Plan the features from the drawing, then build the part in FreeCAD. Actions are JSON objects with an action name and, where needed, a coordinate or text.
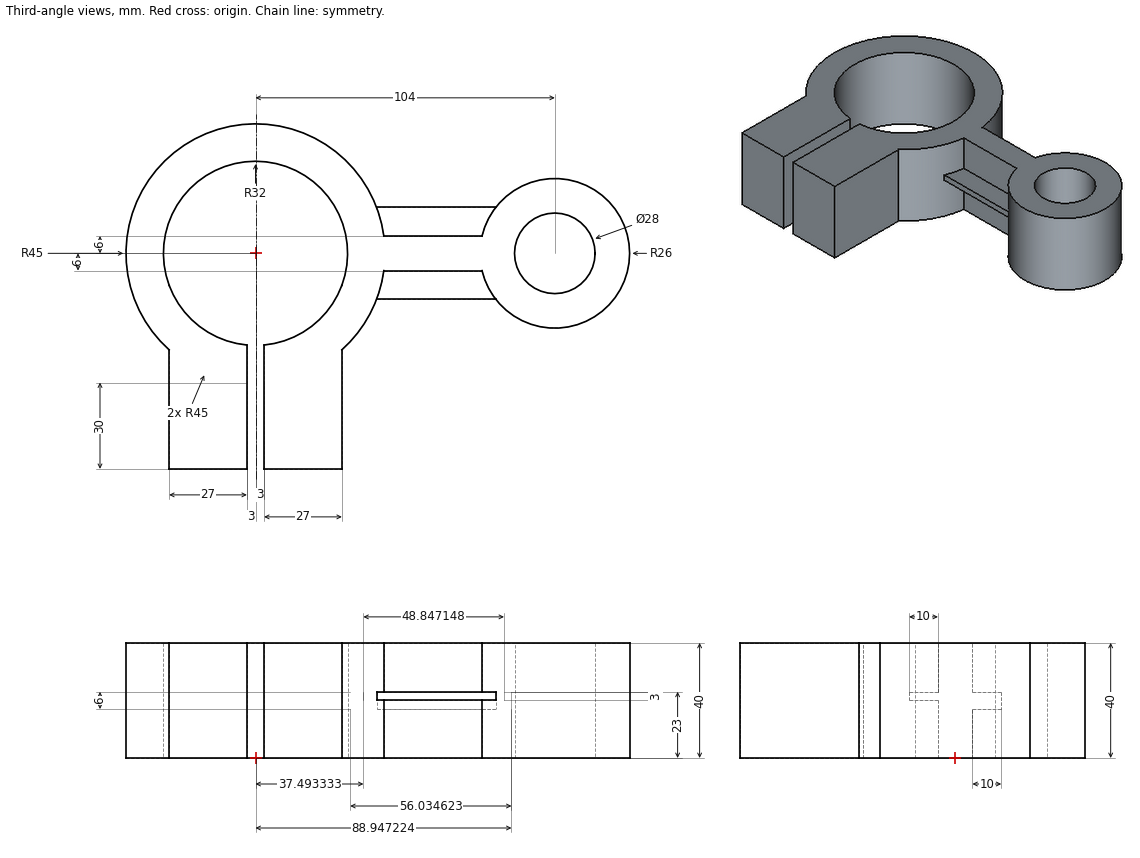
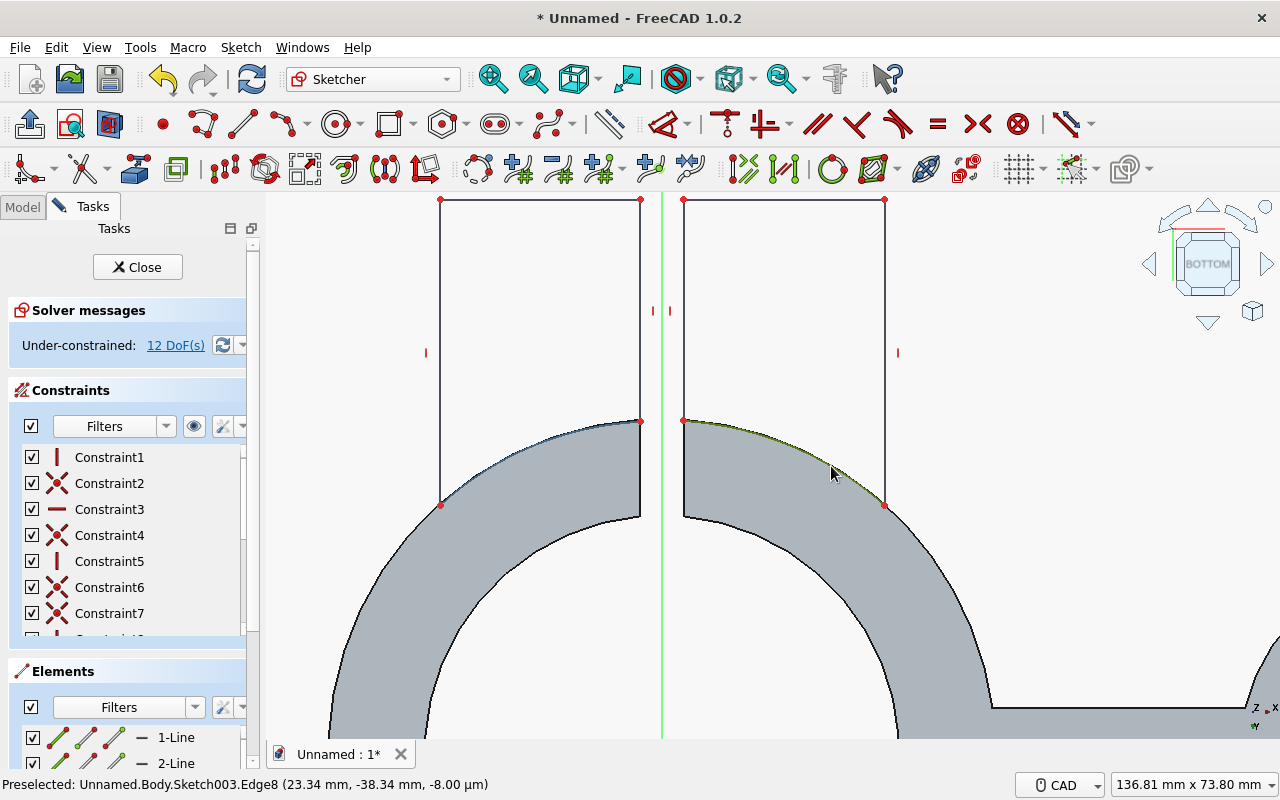
{"action": "left_click", "coordinate": [726, 124]}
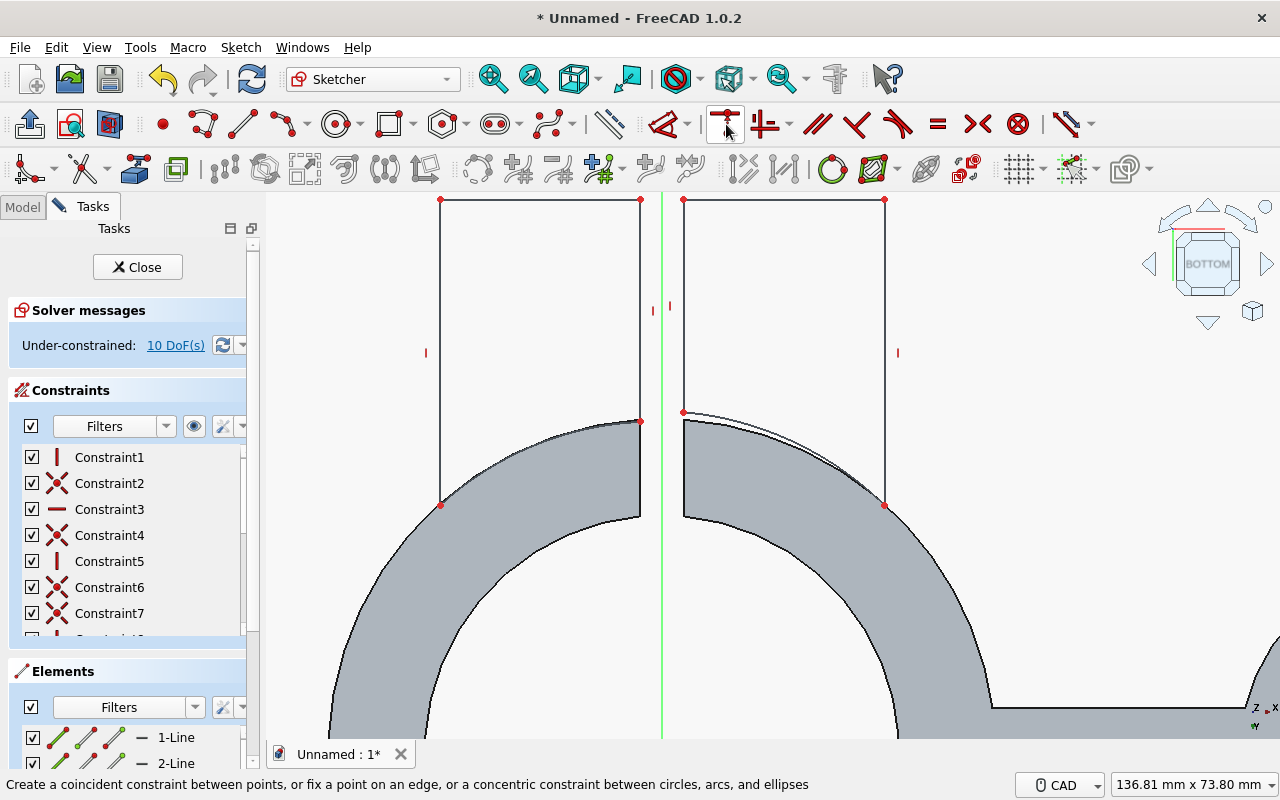
{"action": "scroll", "coordinate": [791, 446], "scroll_direction": "down", "scroll_amount": 2}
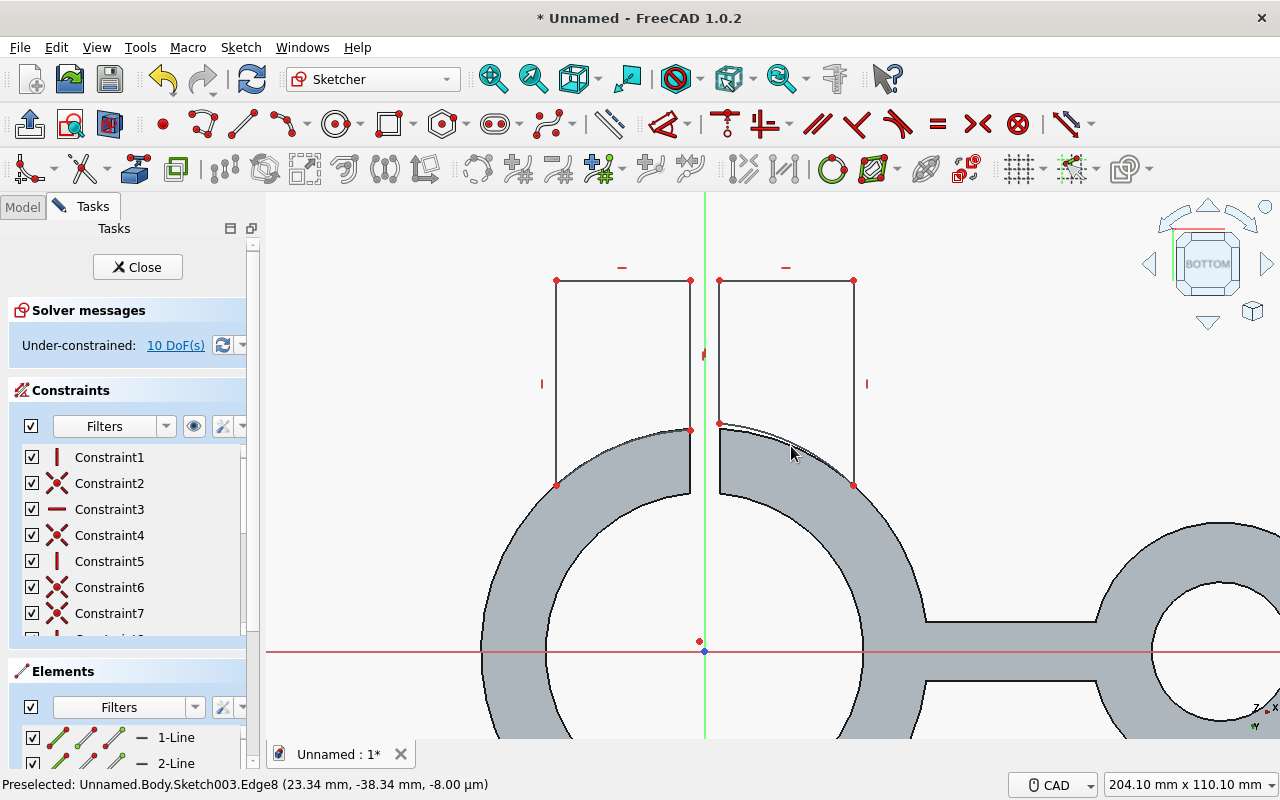
{"action": "left_click_drag", "start_coordinate": [690, 632], "coordinate": [715, 662]}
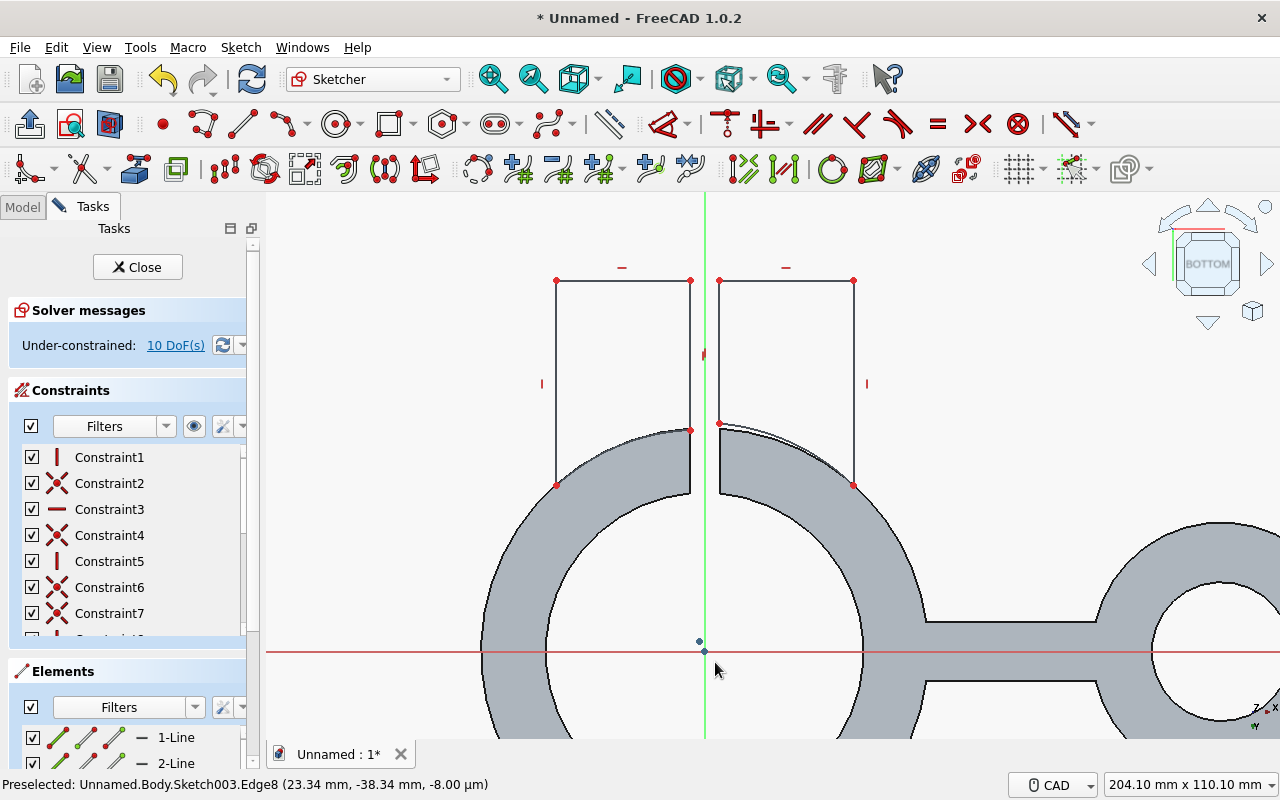
{"action": "key", "text": "c"}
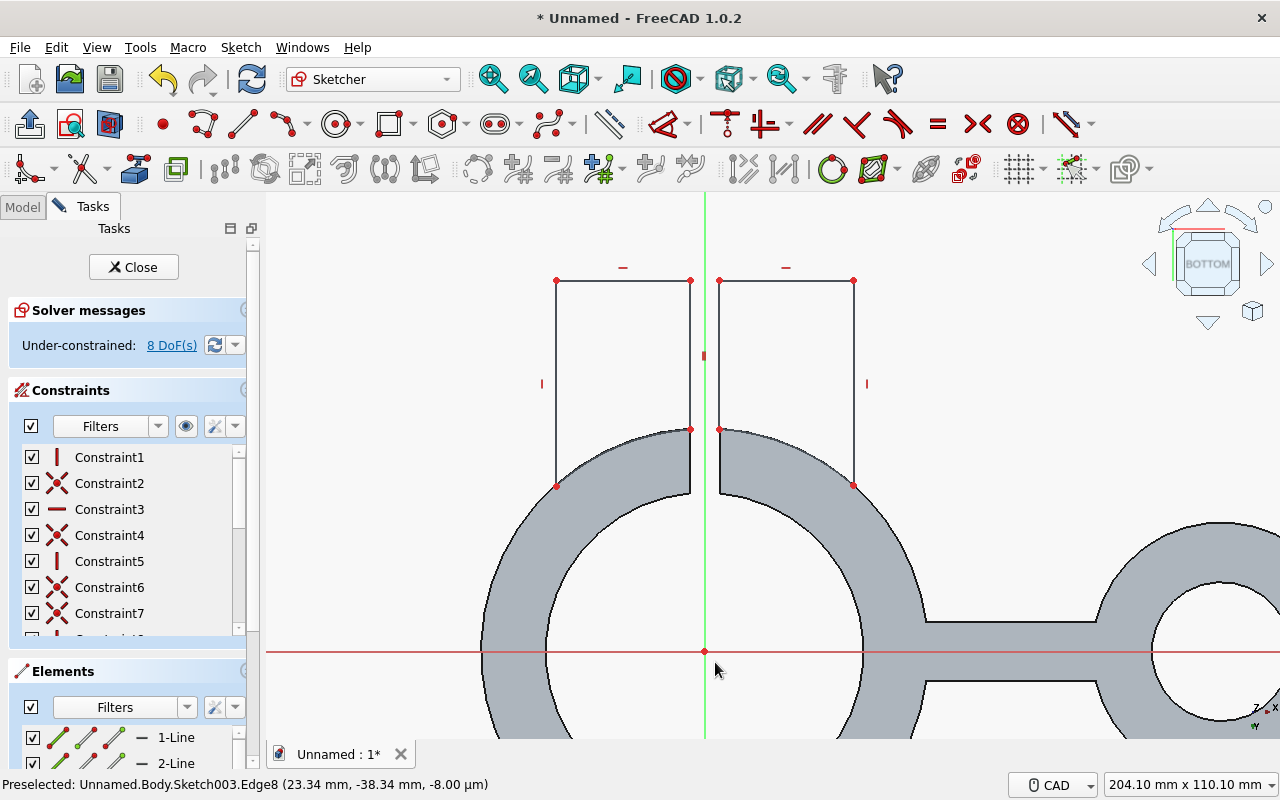
{"action": "left_click", "coordinate": [646, 437]}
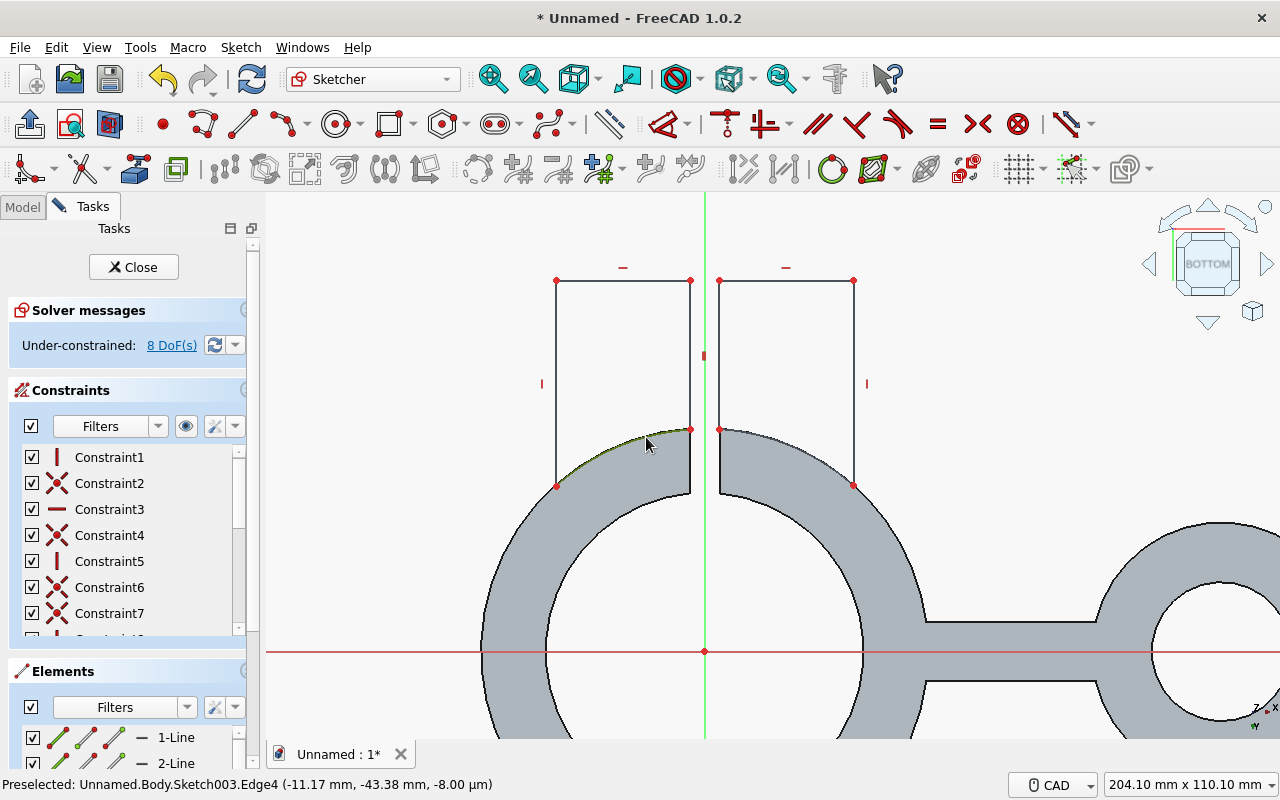
{"action": "left_click", "coordinate": [818, 460]}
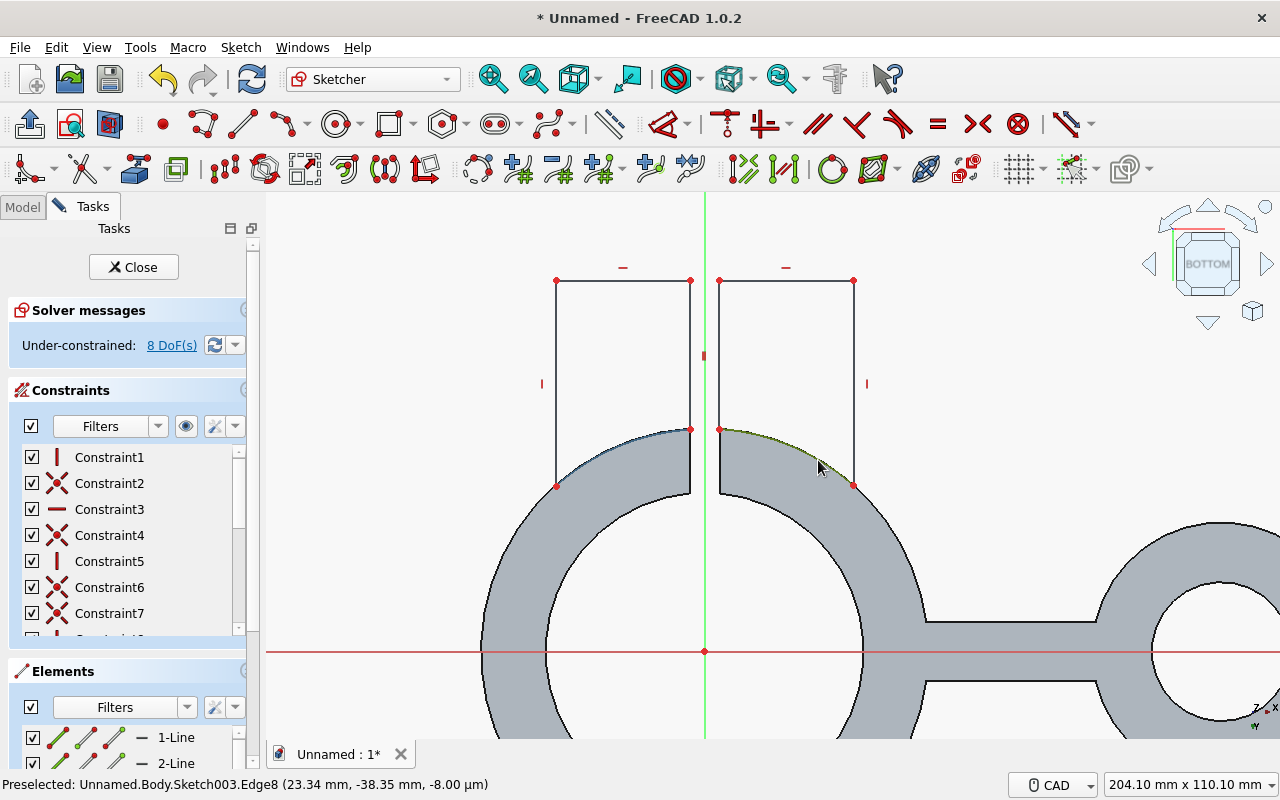
{"action": "key", "text": "e"}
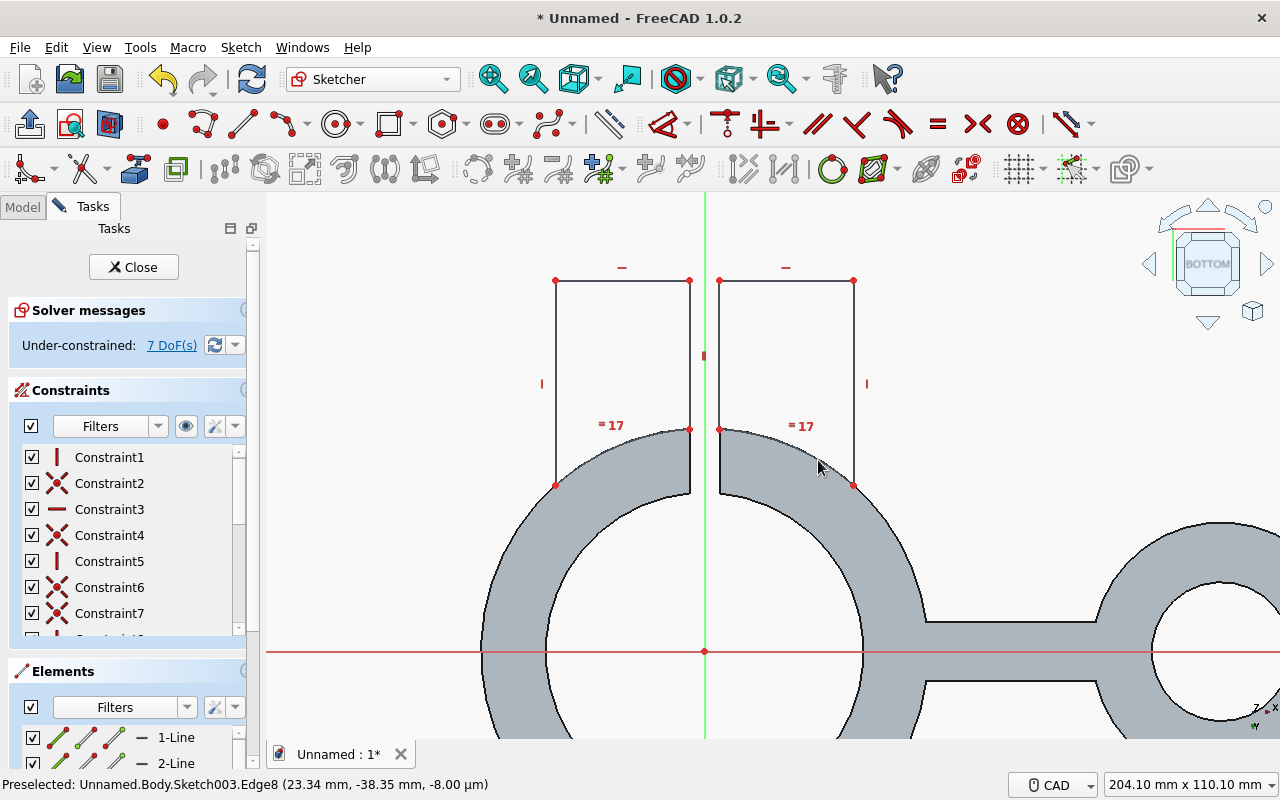
{"action": "left_click", "coordinate": [690, 281]}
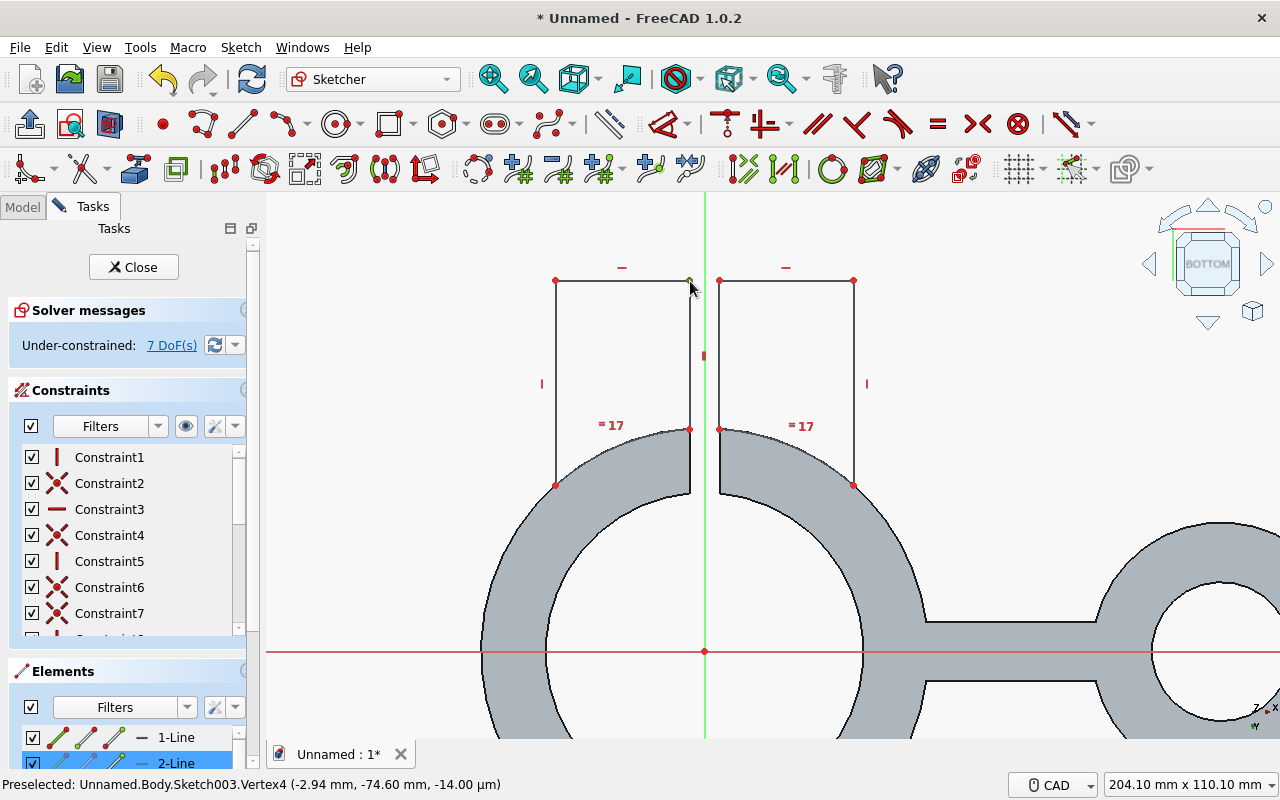
{"action": "left_click", "coordinate": [719, 281]}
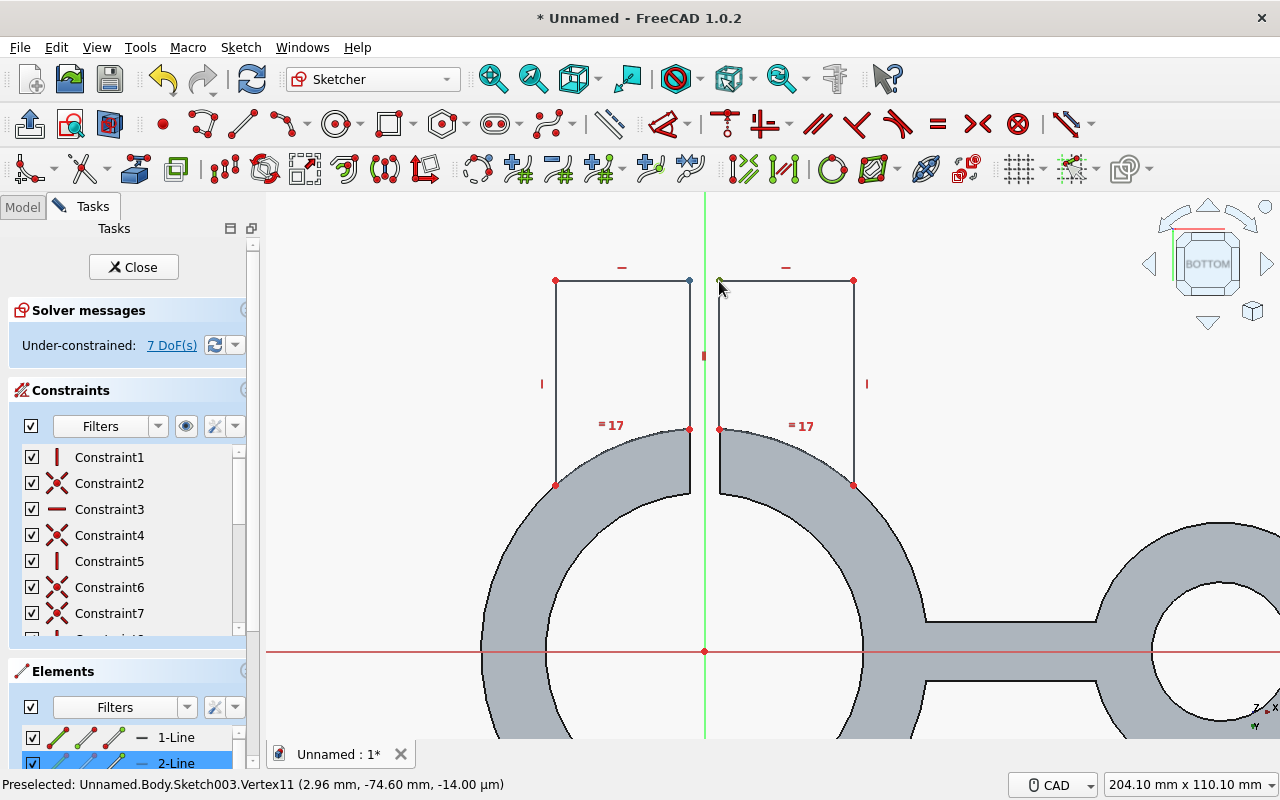
{"action": "left_click", "coordinate": [705, 606]}